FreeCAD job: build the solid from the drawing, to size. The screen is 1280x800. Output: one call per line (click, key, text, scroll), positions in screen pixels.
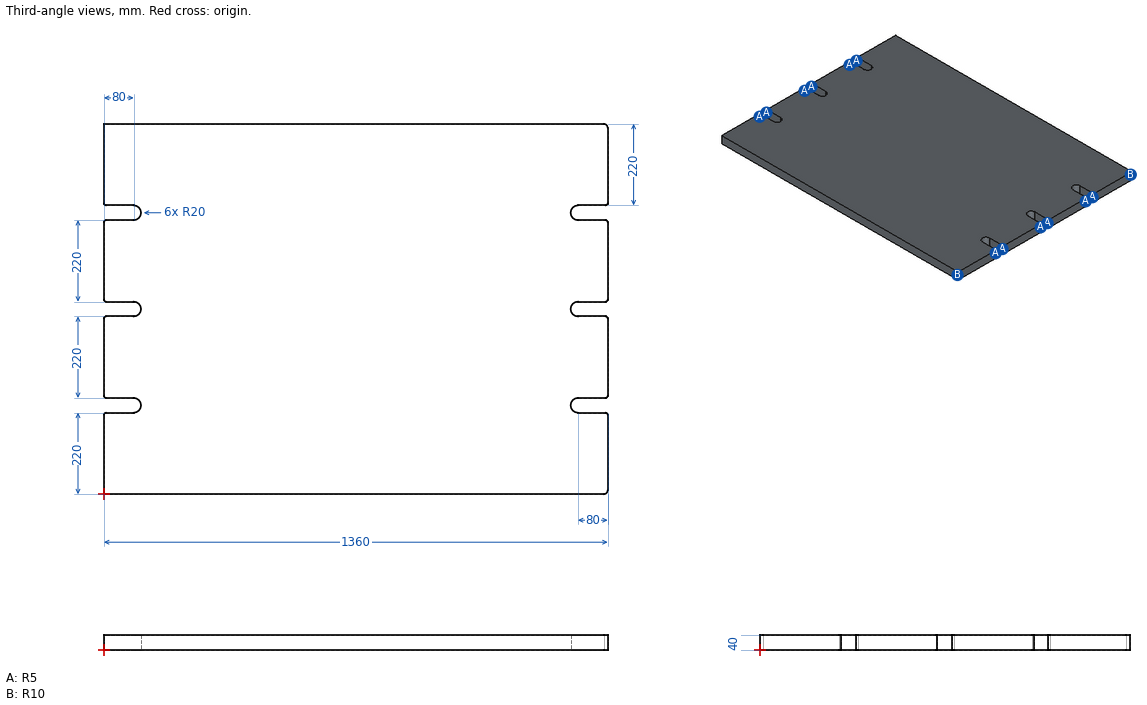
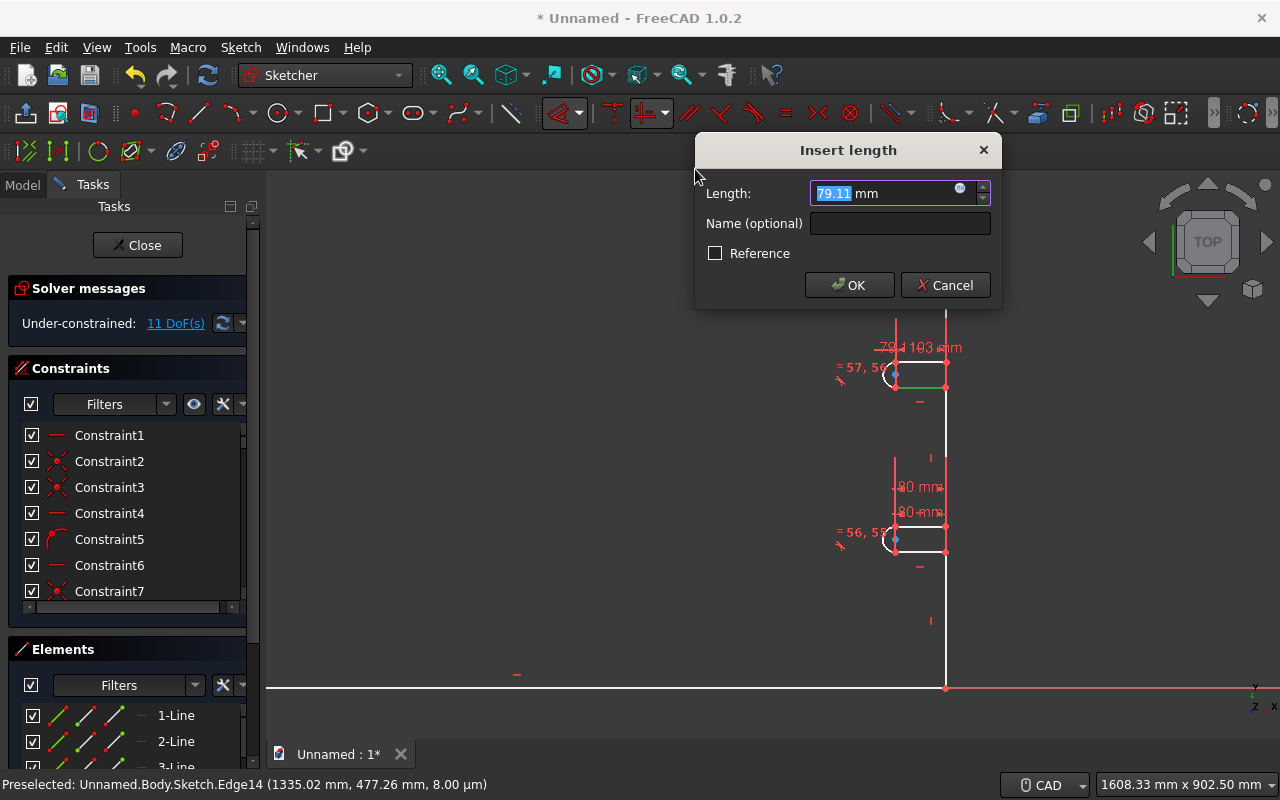
text(80)
key(Return)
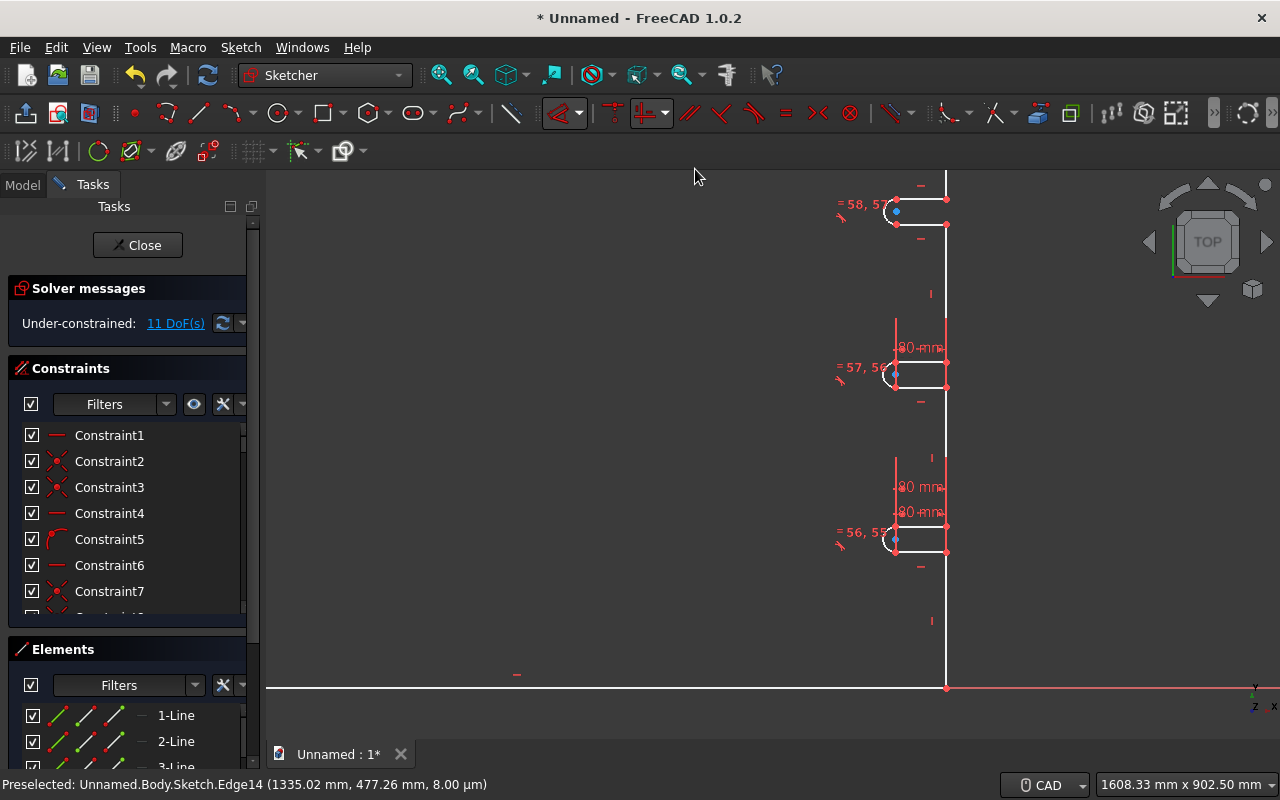
click(911, 362)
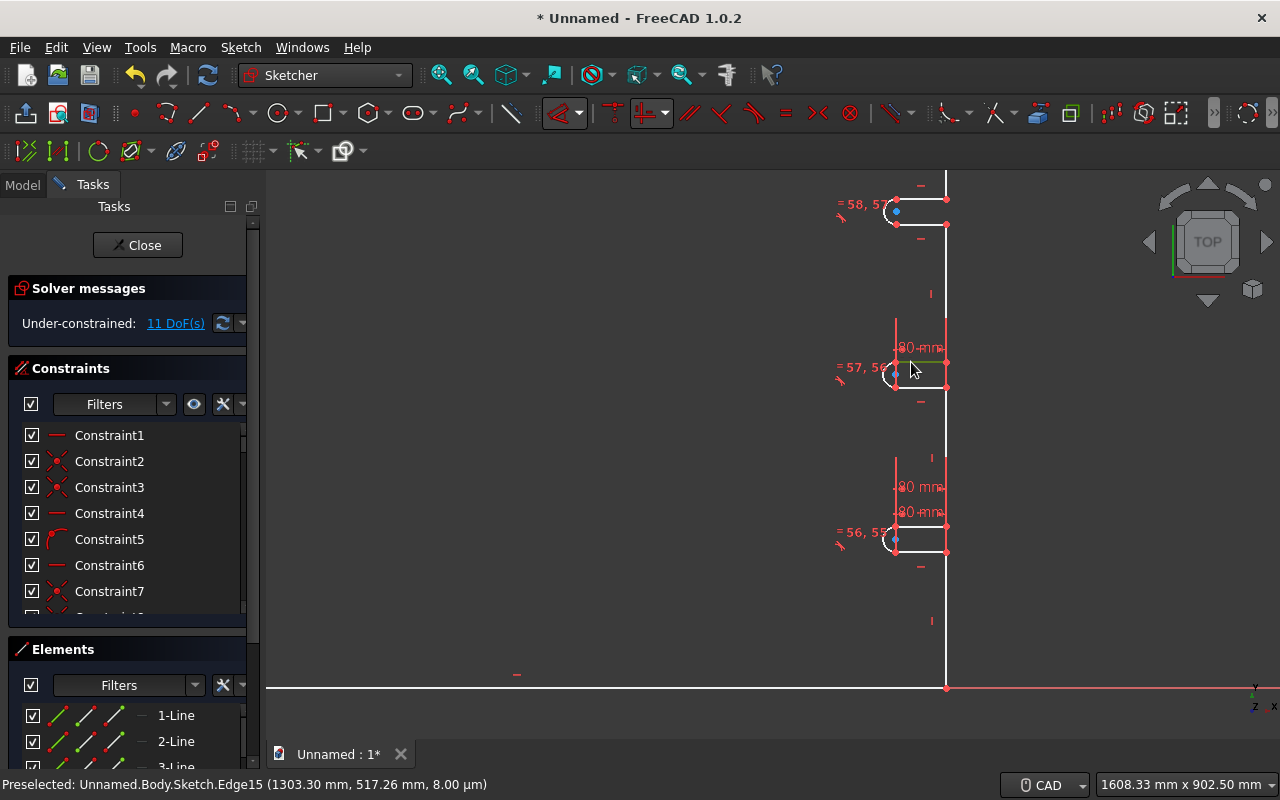
click(582, 114)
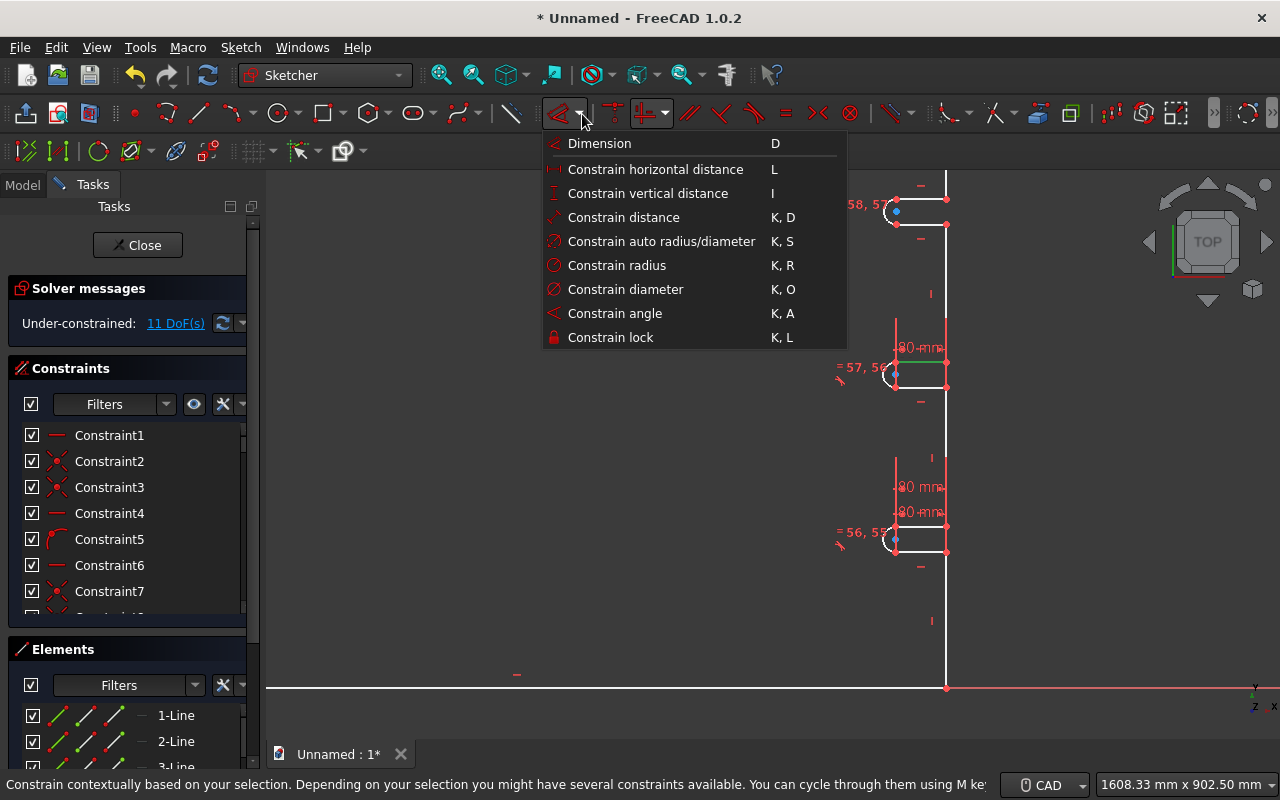
click(695, 169)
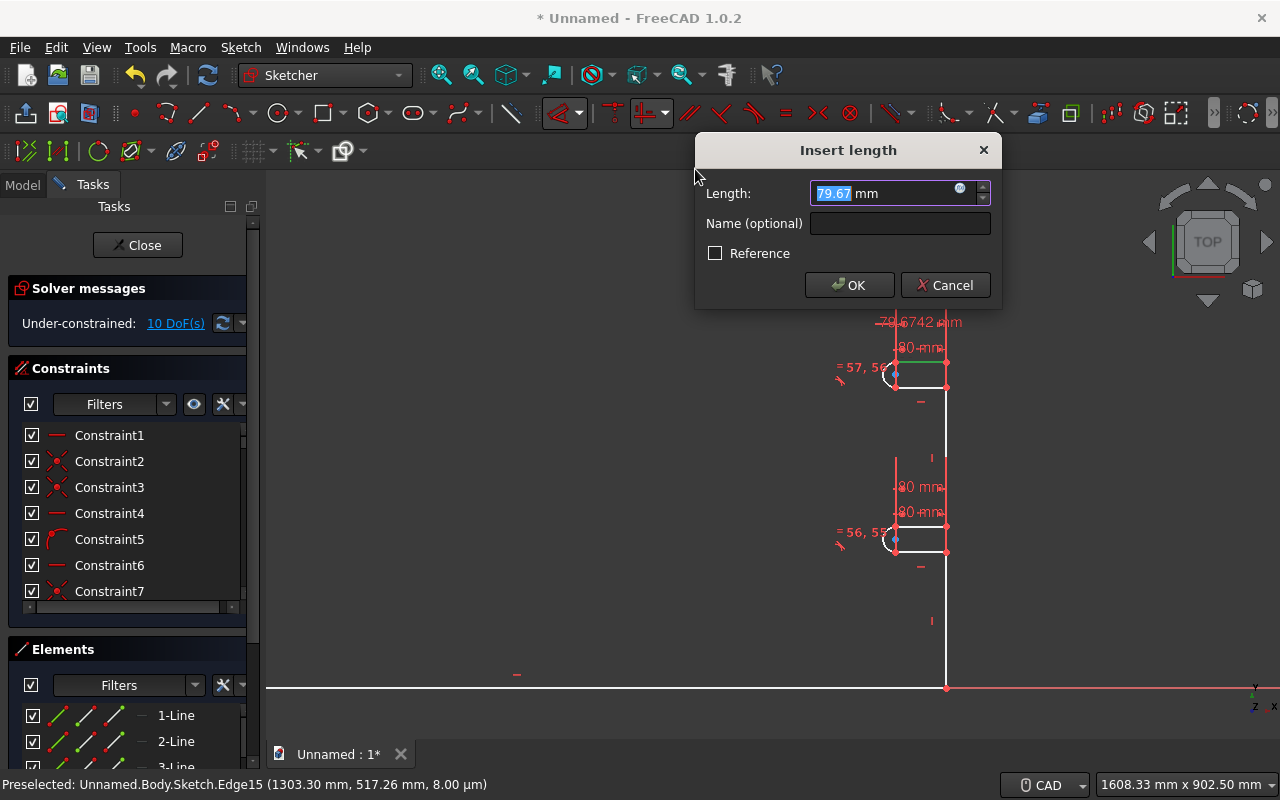
text(80)
key(Return)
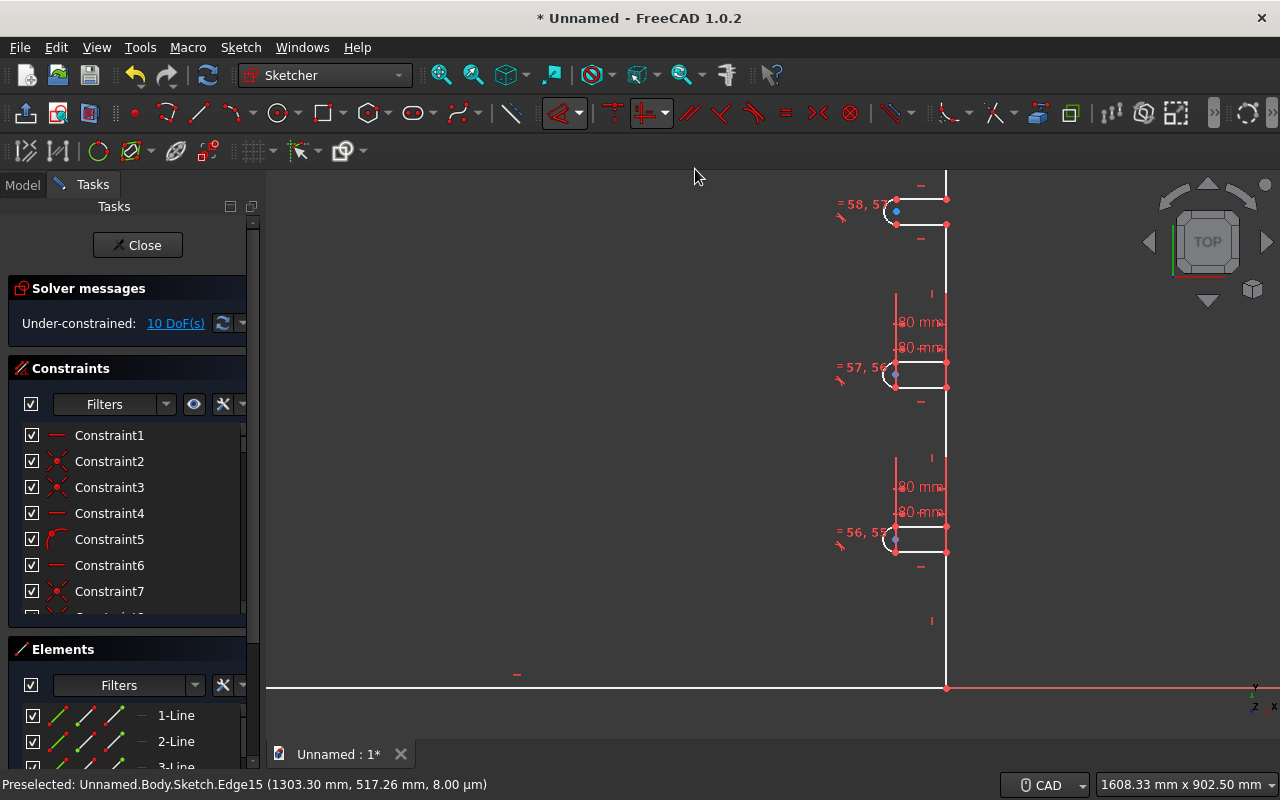
click(931, 225)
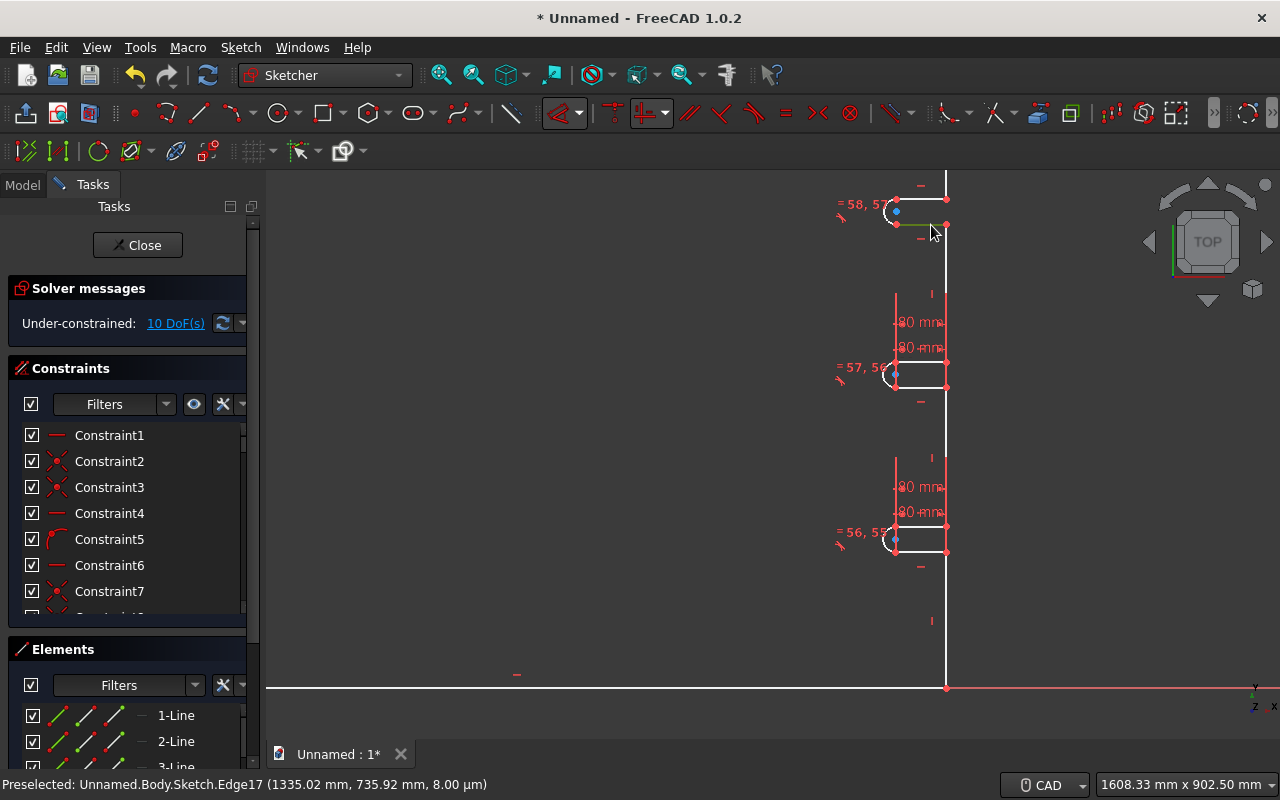
click(582, 114)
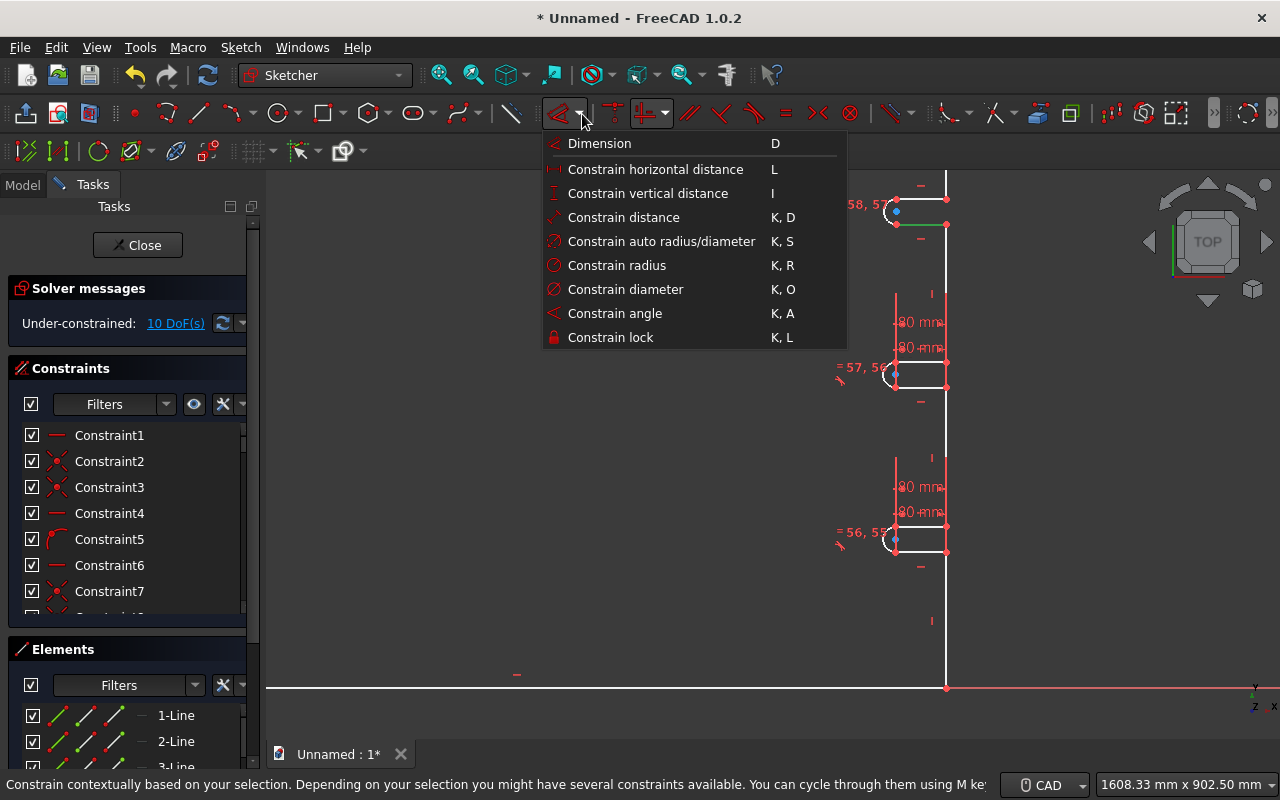
click(695, 169)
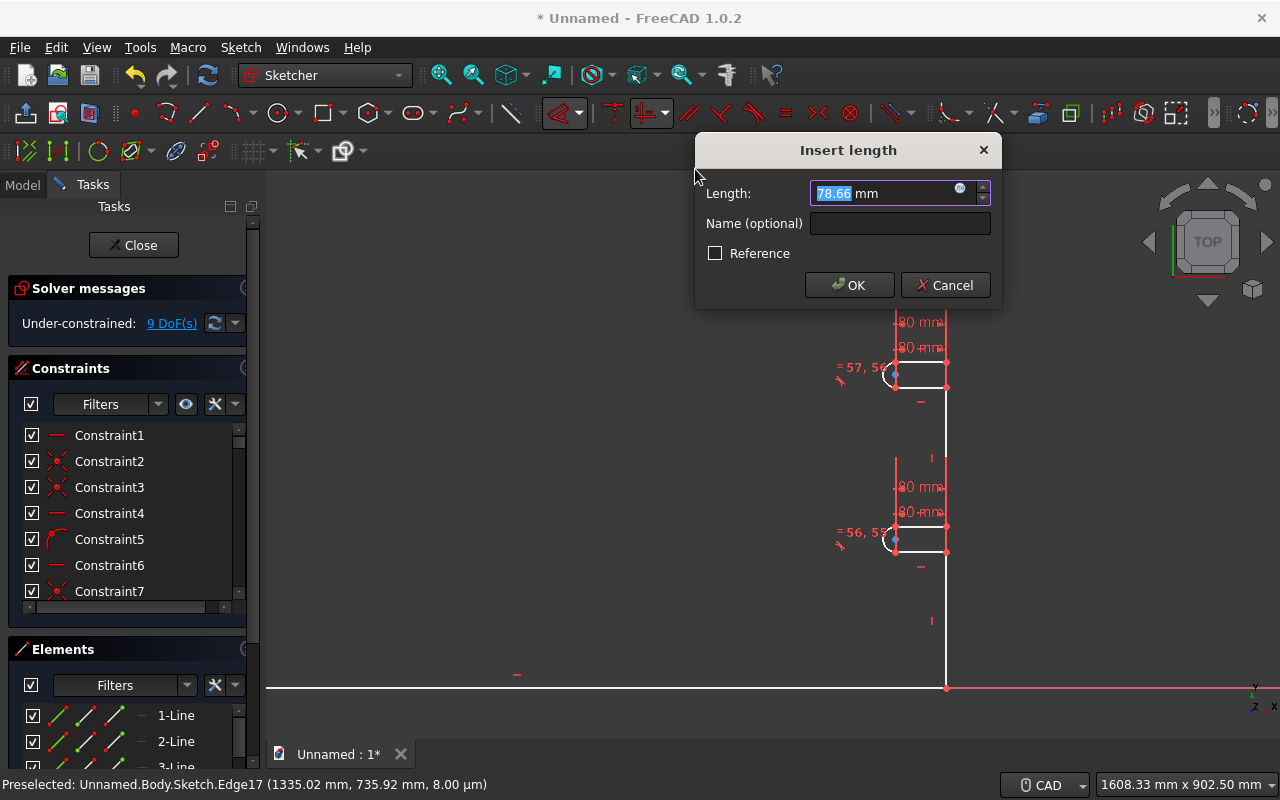
text(80)
key(Return)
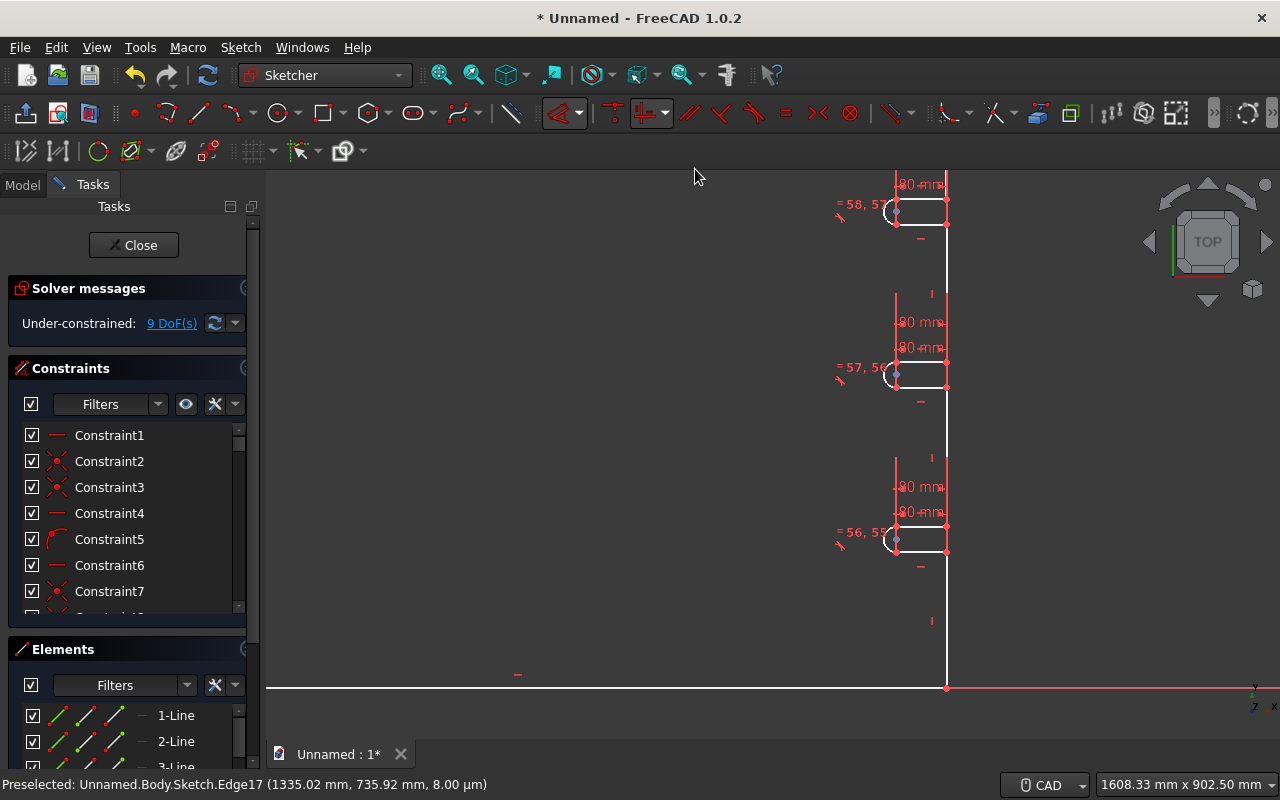
click(911, 199)